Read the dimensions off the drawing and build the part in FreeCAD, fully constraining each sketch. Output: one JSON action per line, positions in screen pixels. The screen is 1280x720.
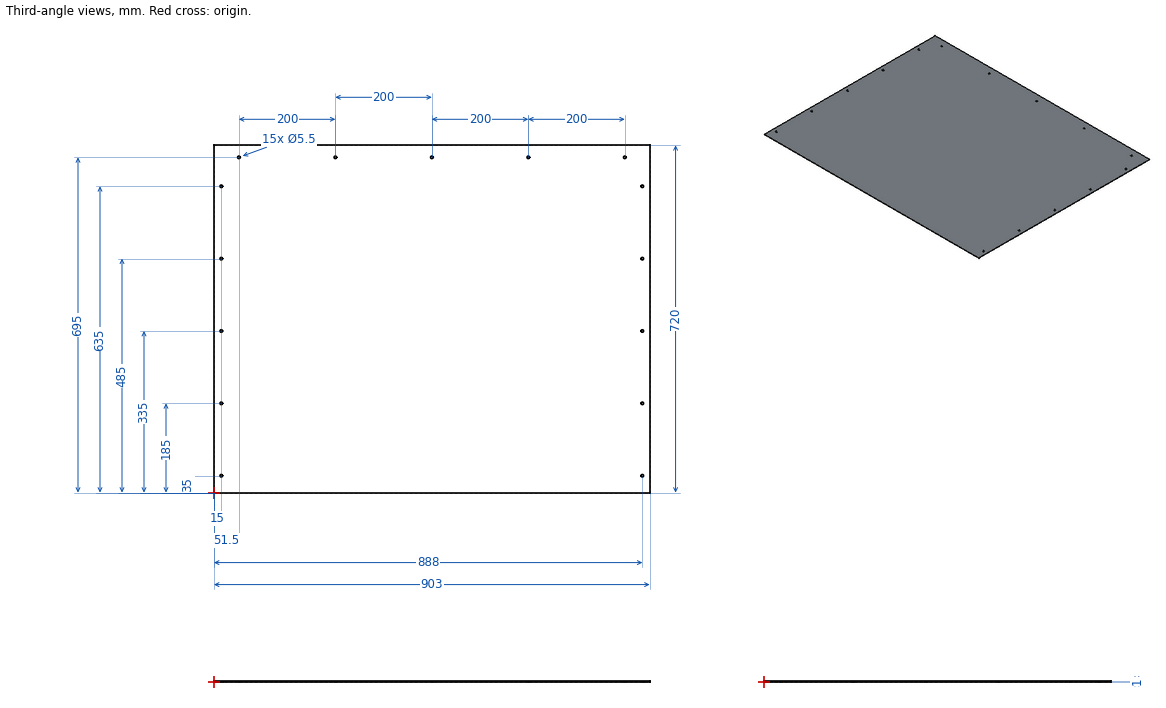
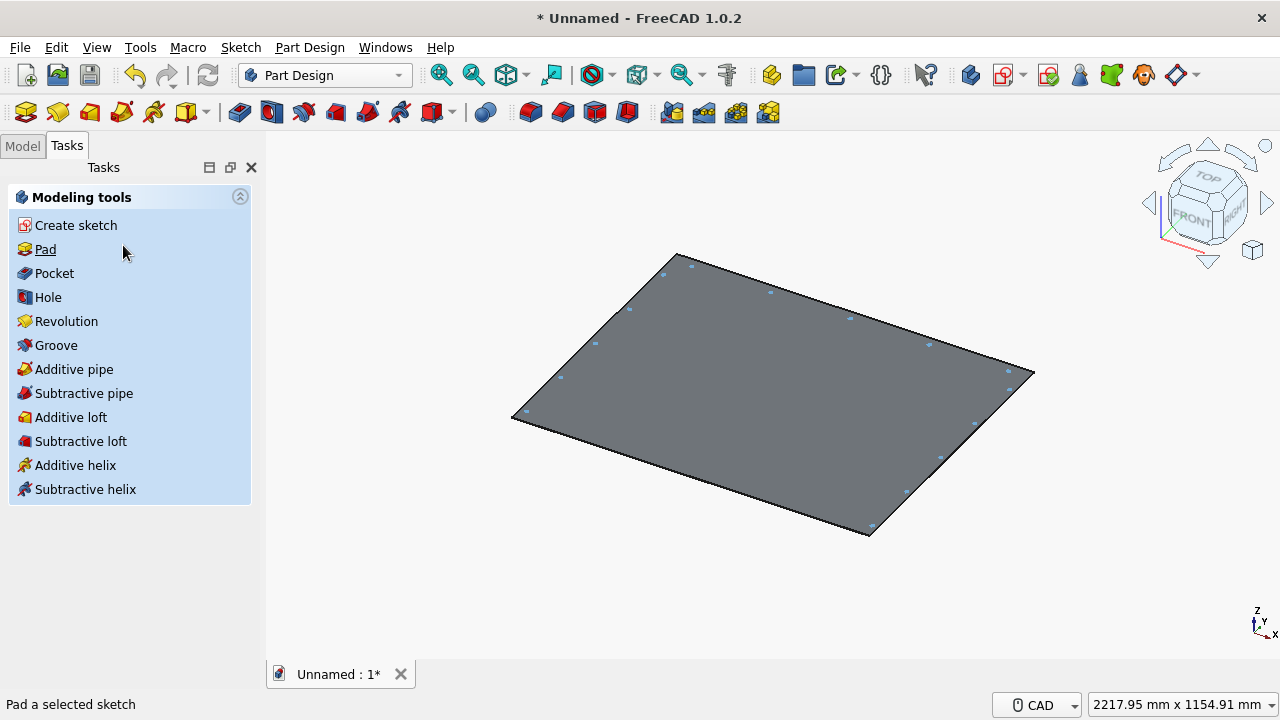
{"action": "left_click", "coordinate": [240, 112]}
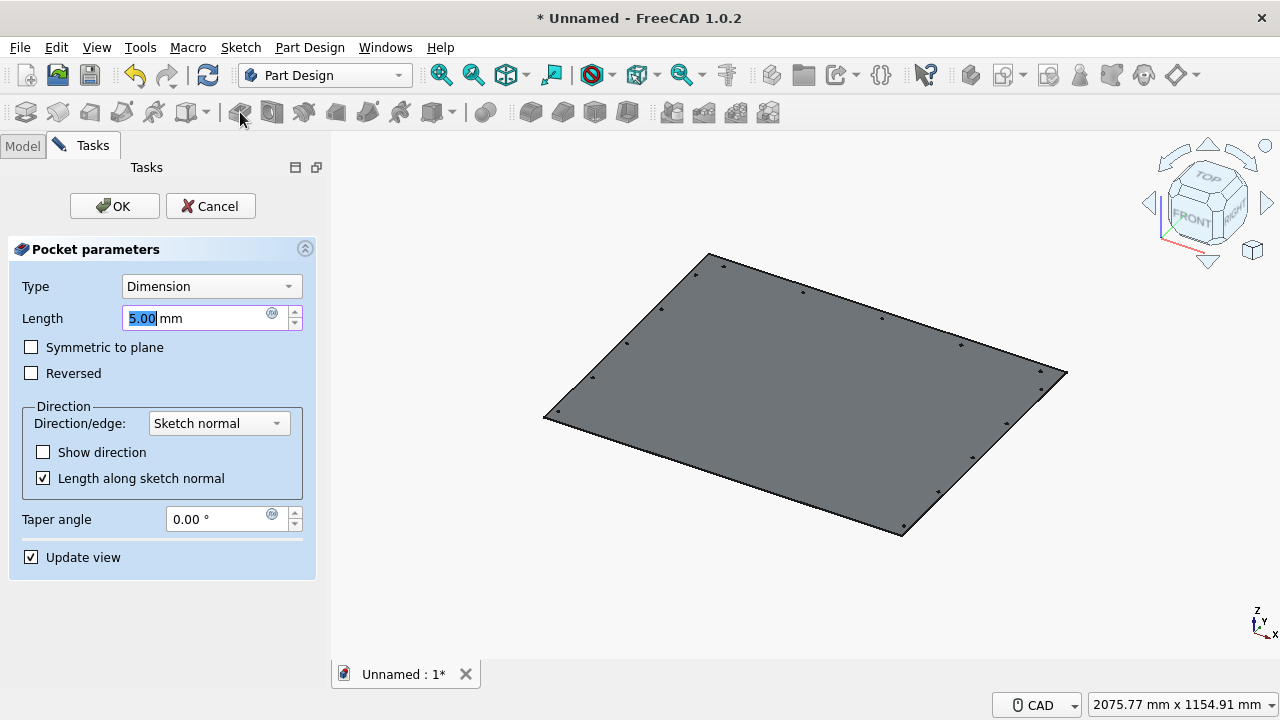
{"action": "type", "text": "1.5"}
{"action": "key", "text": "Tab"}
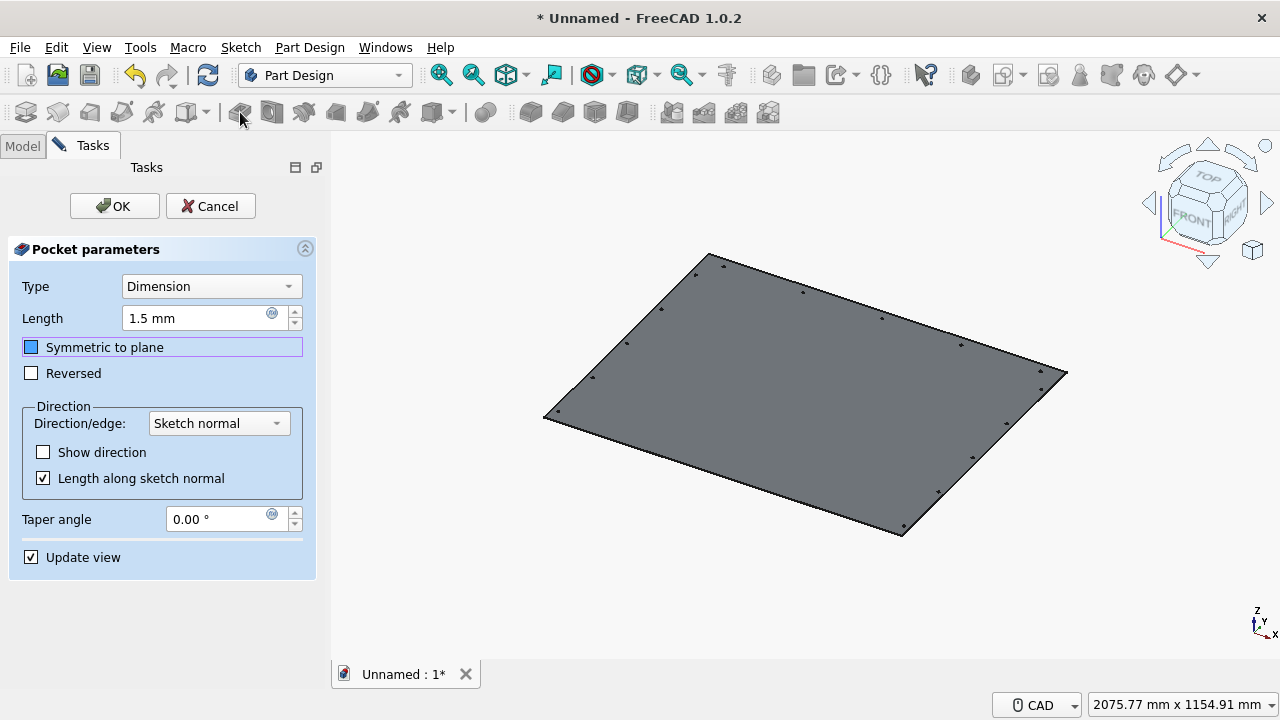
{"action": "left_click", "coordinate": [115, 206]}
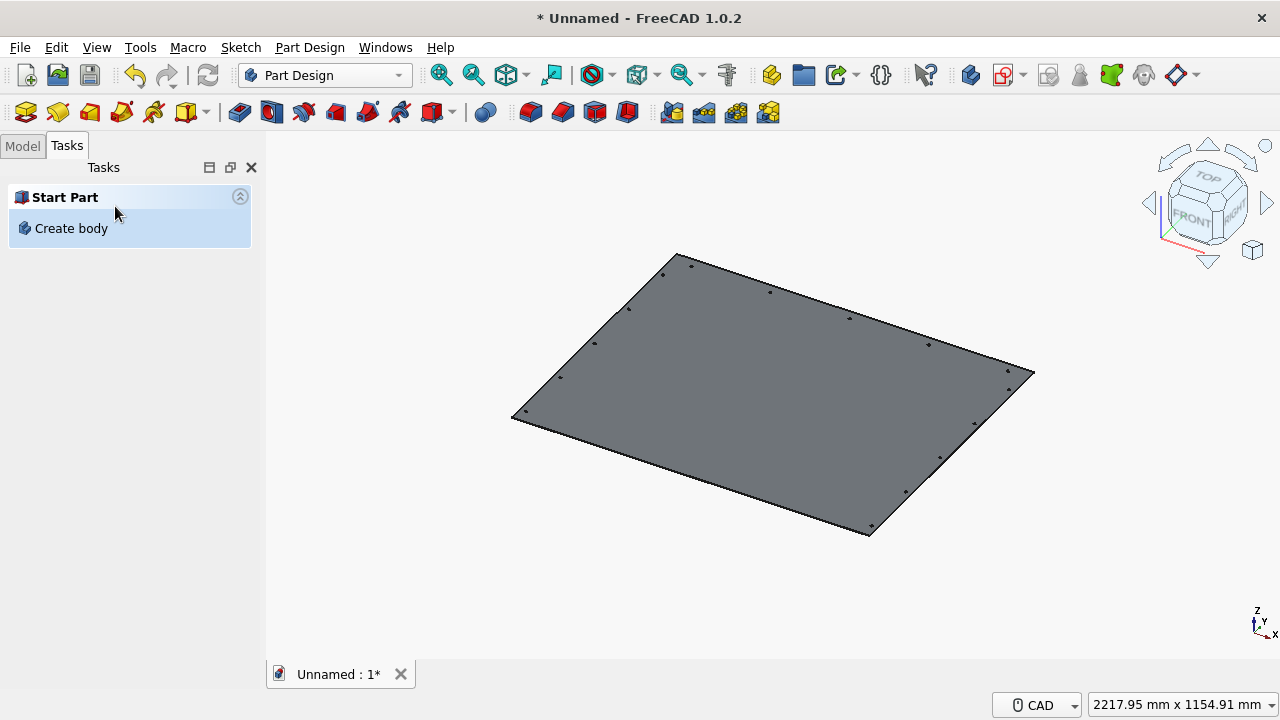
{"action": "key", "text": "0"}